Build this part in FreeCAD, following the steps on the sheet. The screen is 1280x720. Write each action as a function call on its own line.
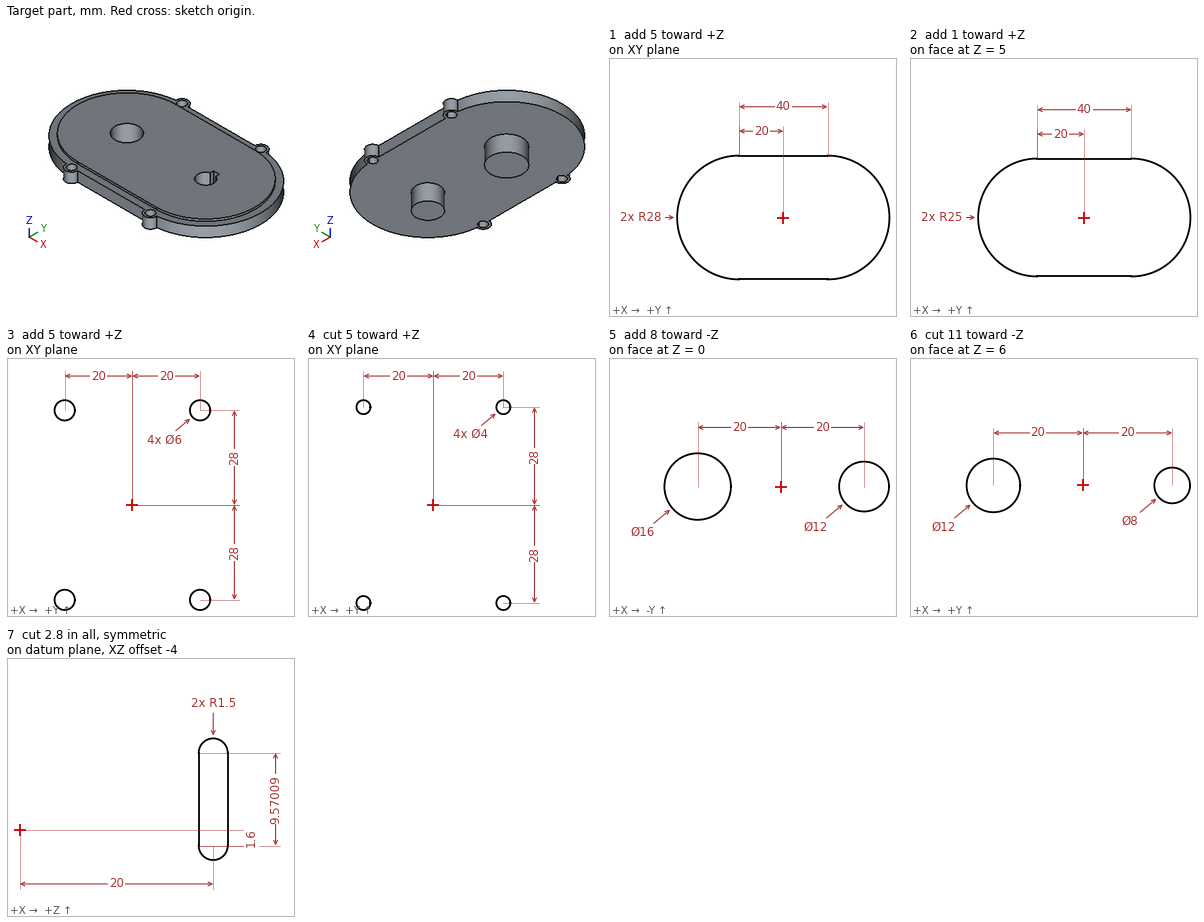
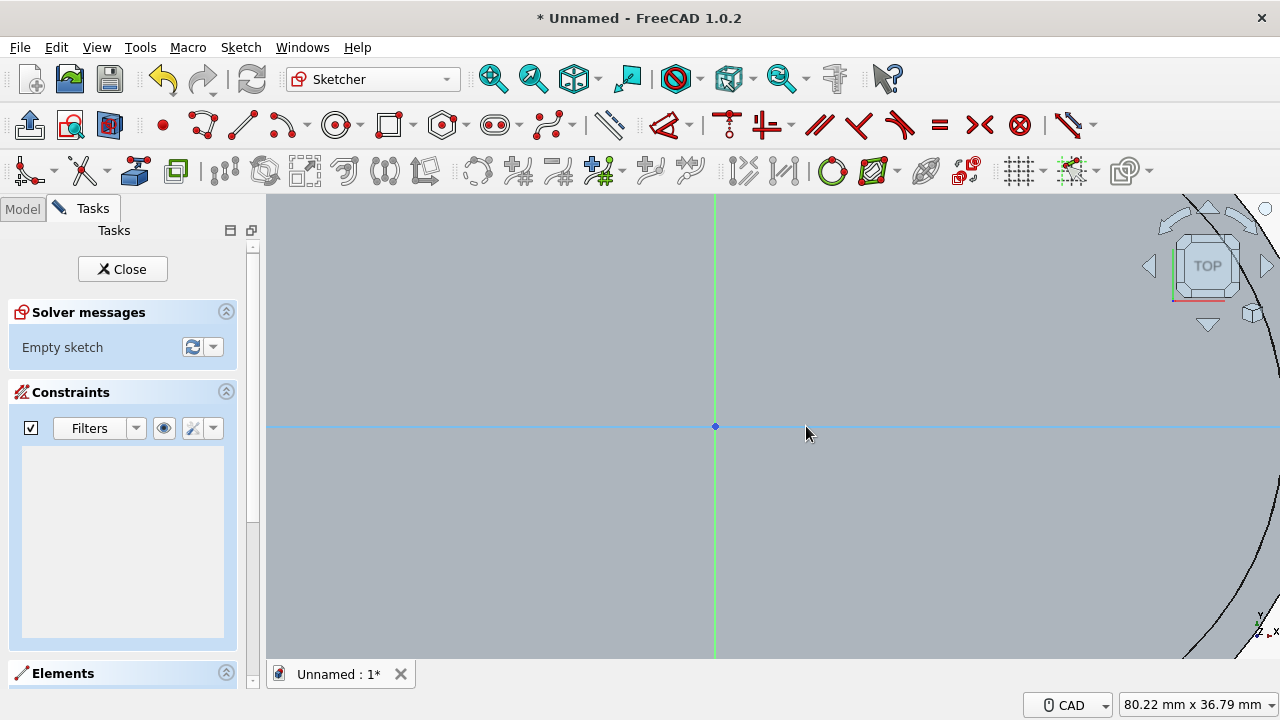
key(g)
key(c)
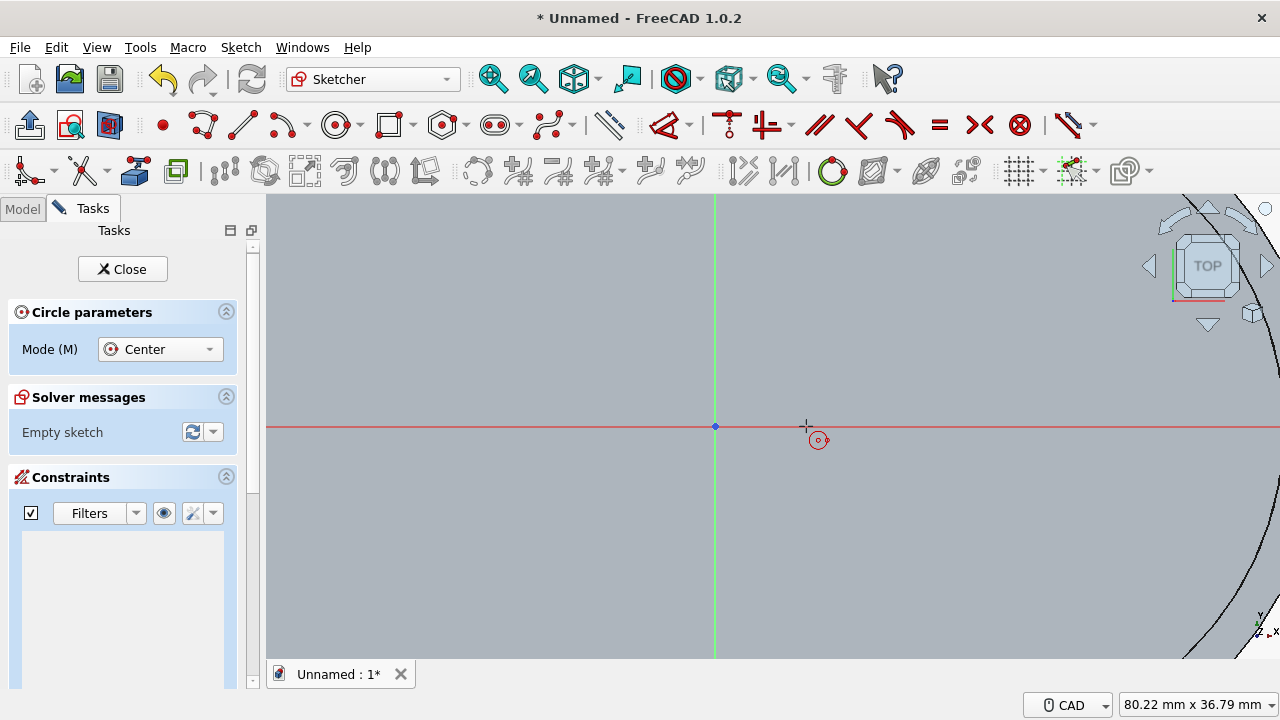
click(463, 426)
click(516, 373)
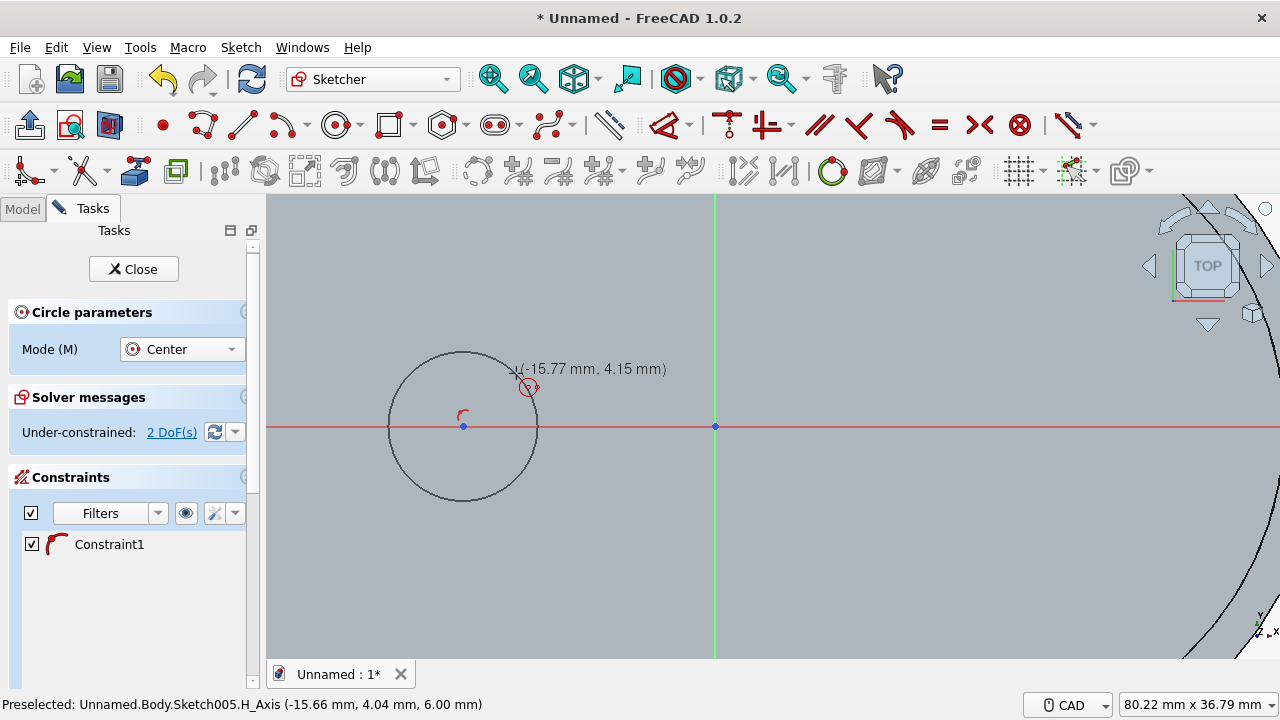
click(968, 426)
click(1004, 391)
key(Escape)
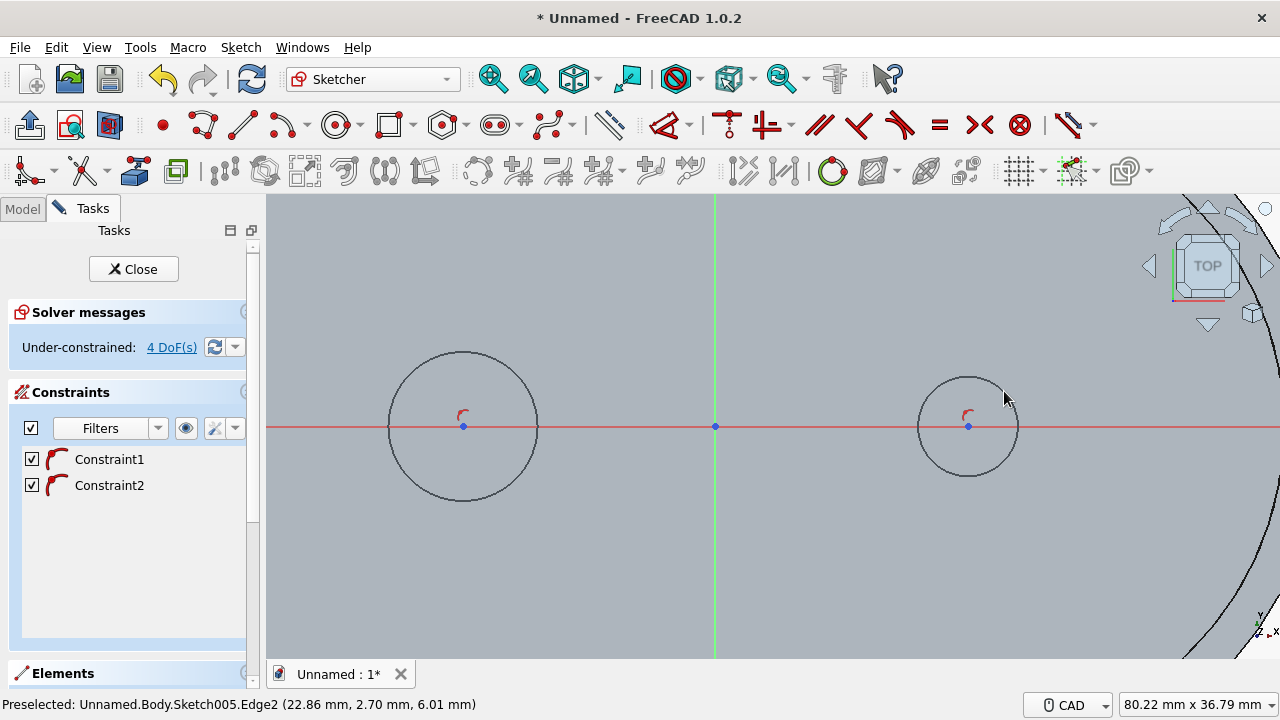
key(d)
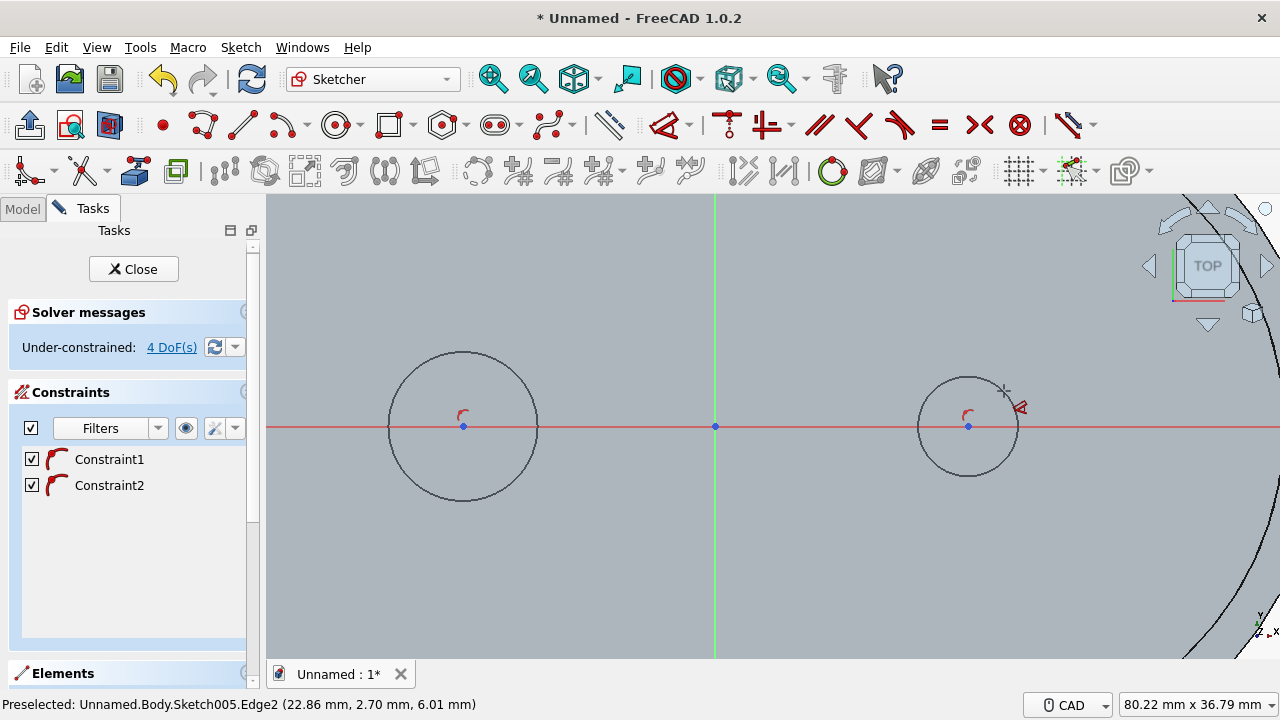
click(516, 374)
click(539, 351)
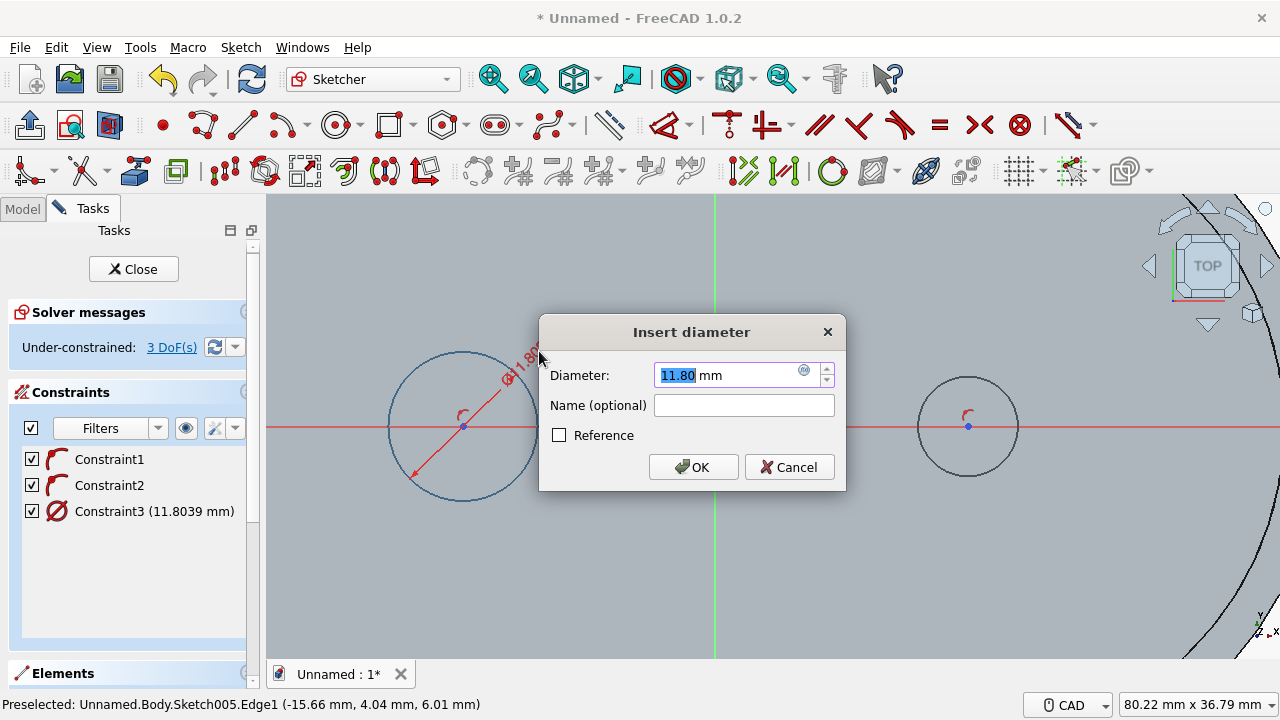
text(12)
key(Return)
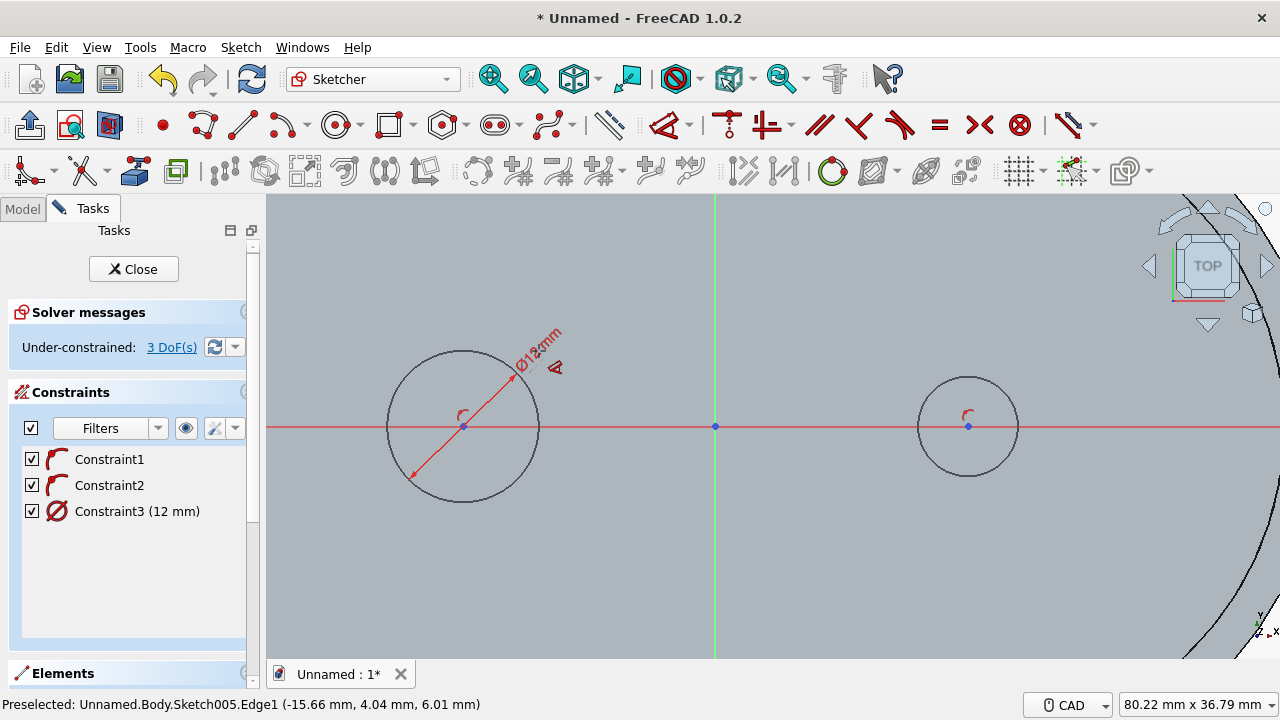
click(1003, 391)
click(1025, 368)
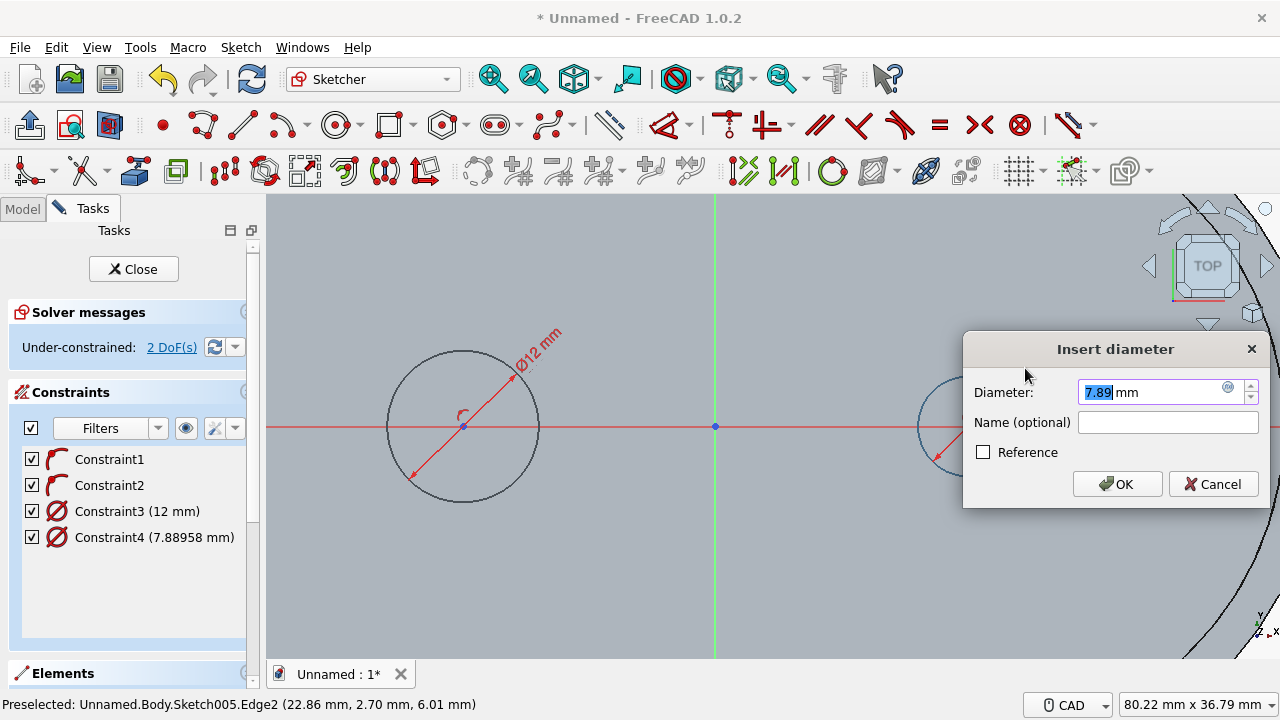
text(8)
key(Return)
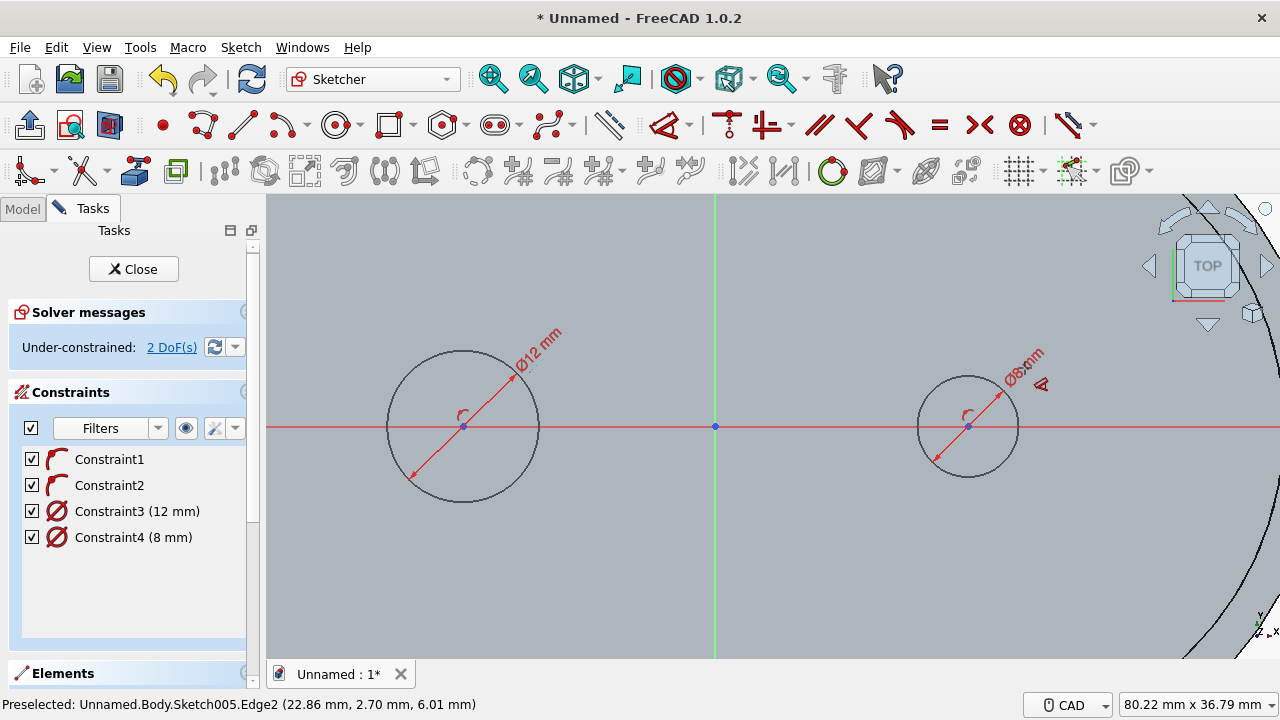
click(463, 426)
click(589, 460)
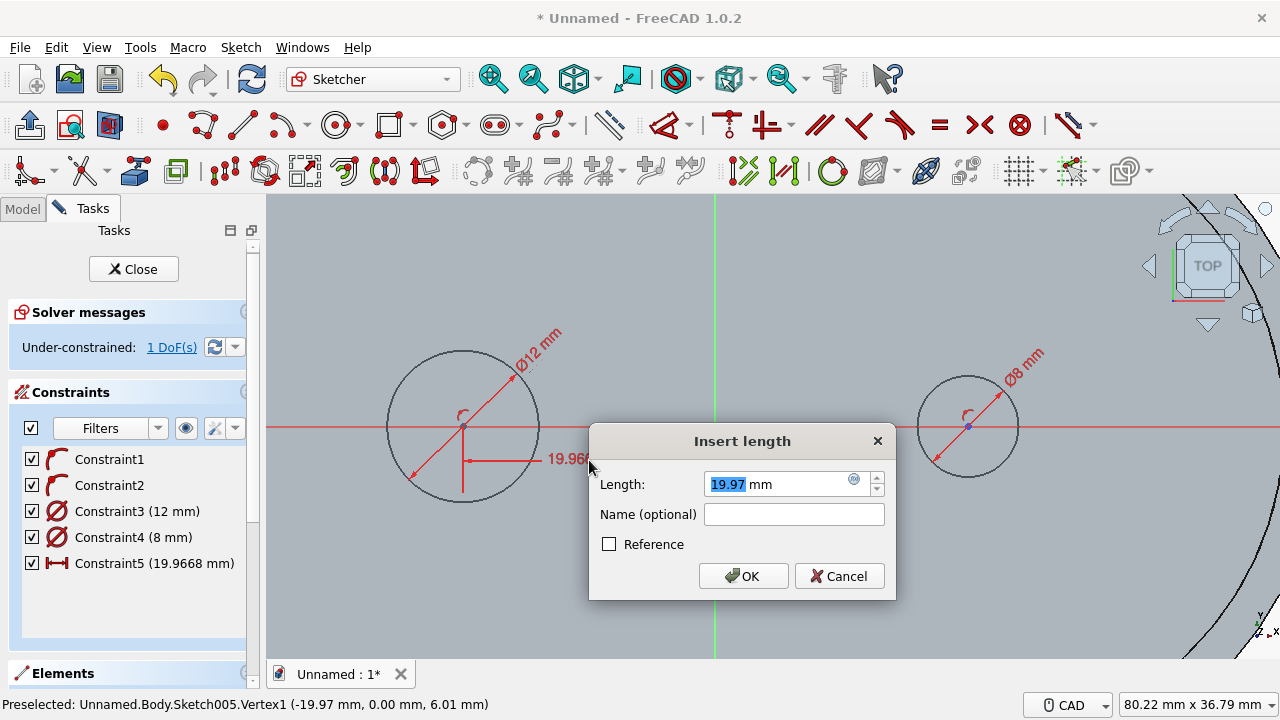
text(20)
key(Return)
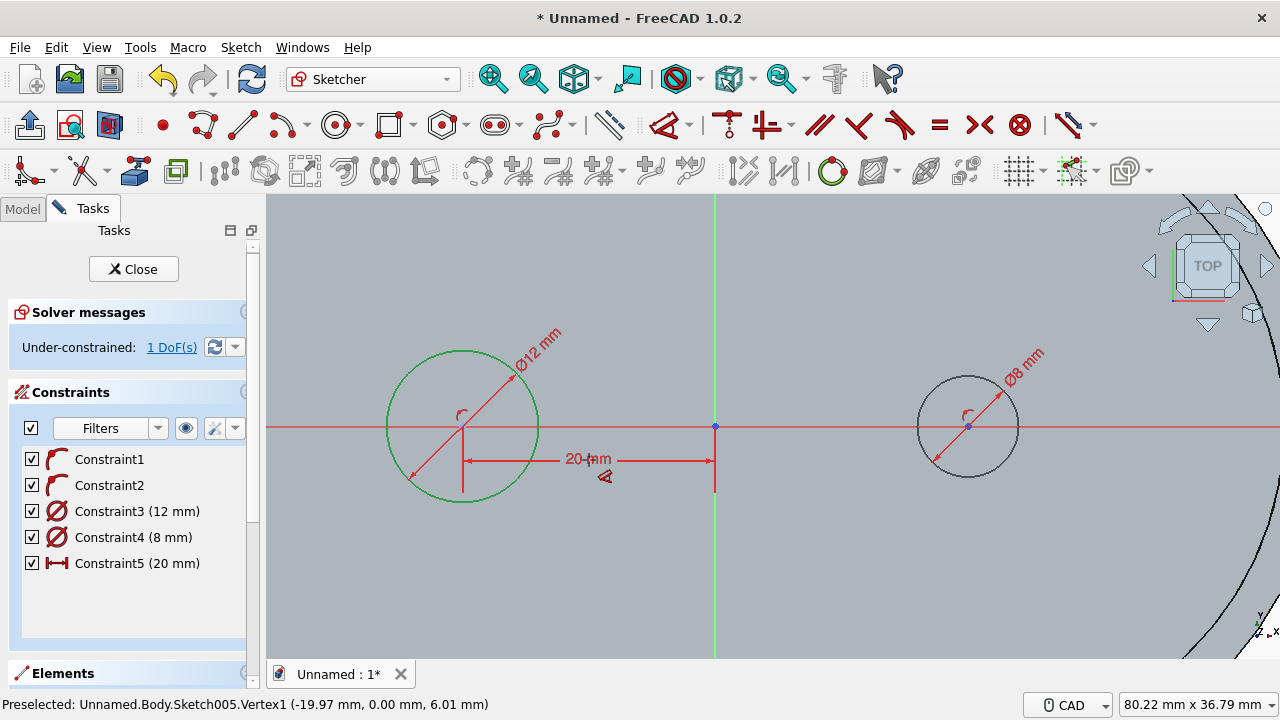
click(968, 426)
click(842, 460)